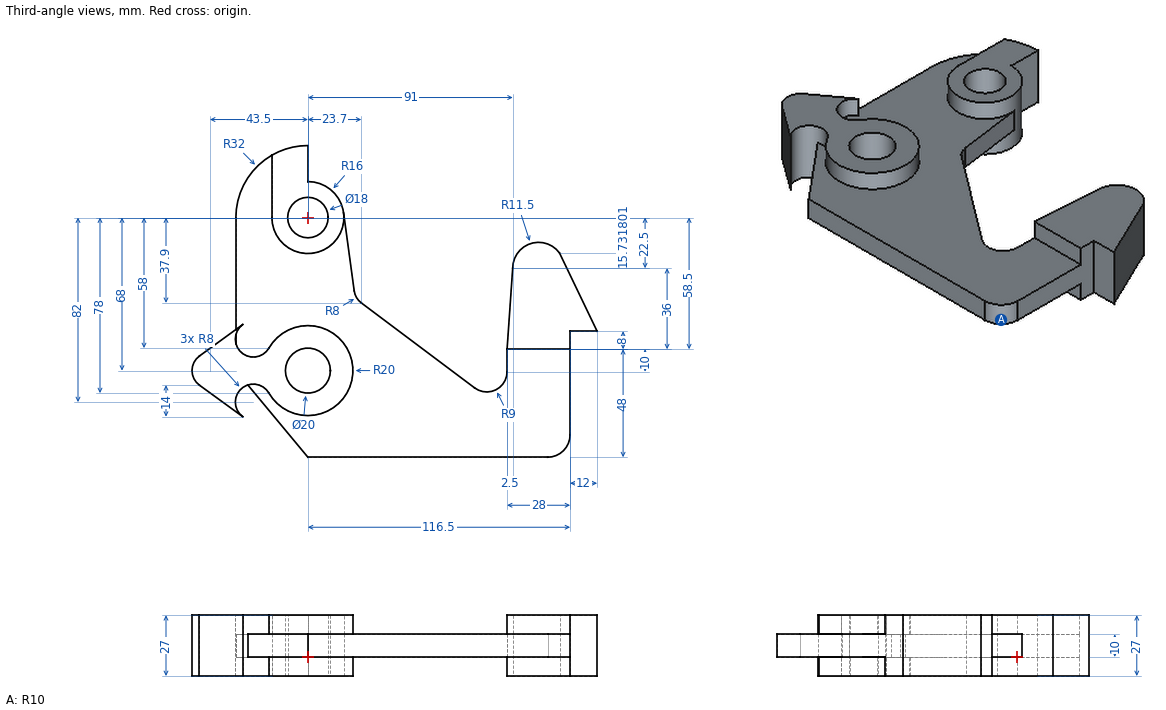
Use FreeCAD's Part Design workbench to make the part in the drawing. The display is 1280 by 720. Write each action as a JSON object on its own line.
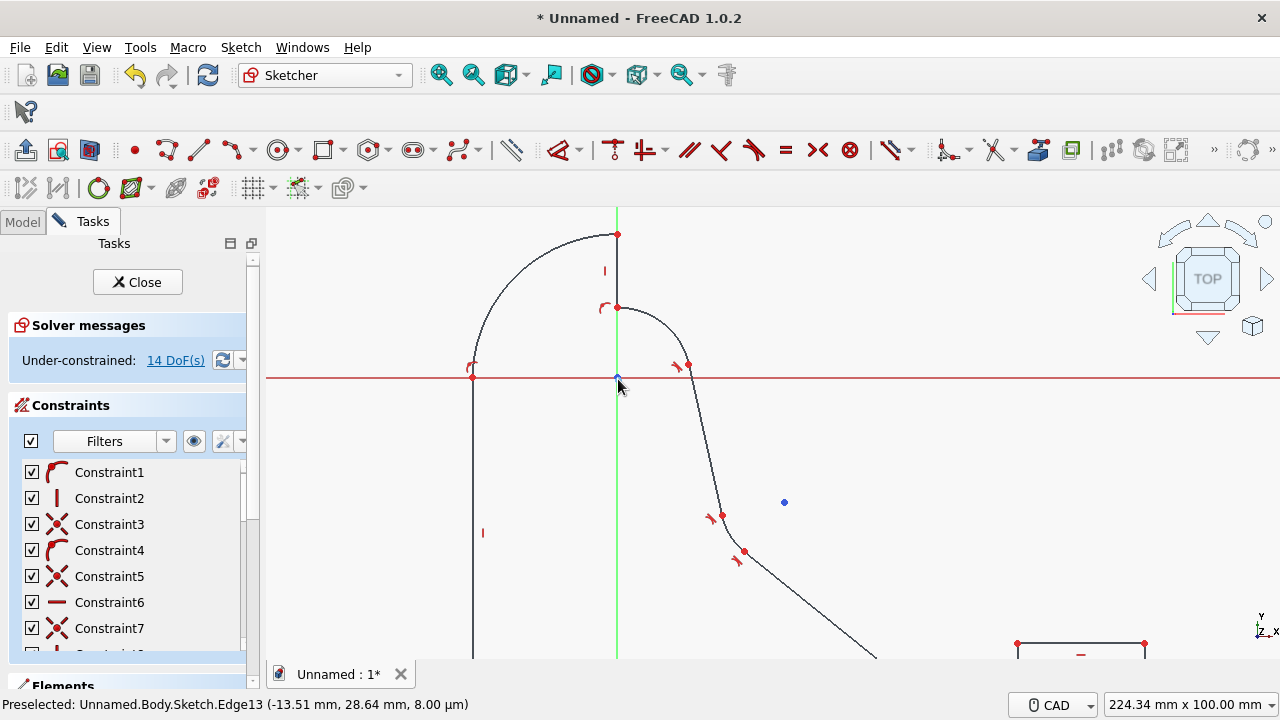
{"action": "left_click_drag", "start_coordinate": [607, 368], "coordinate": [628, 390]}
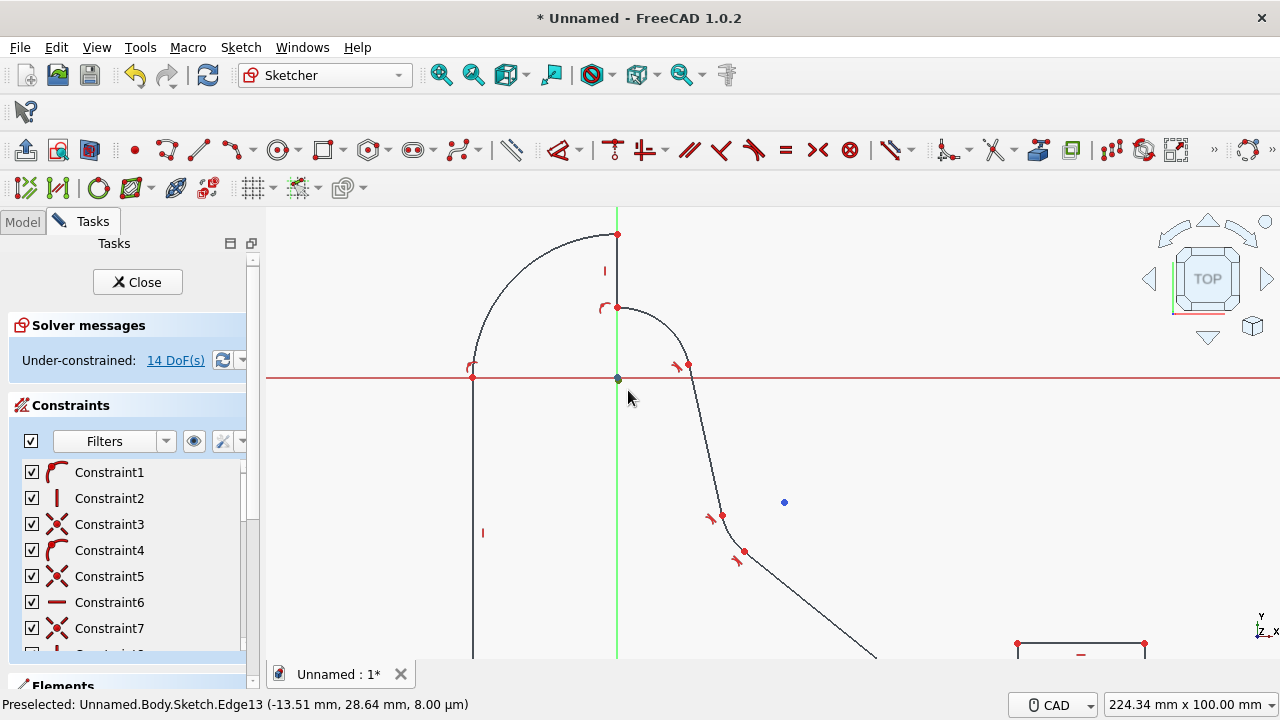
{"action": "left_click", "coordinate": [614, 150]}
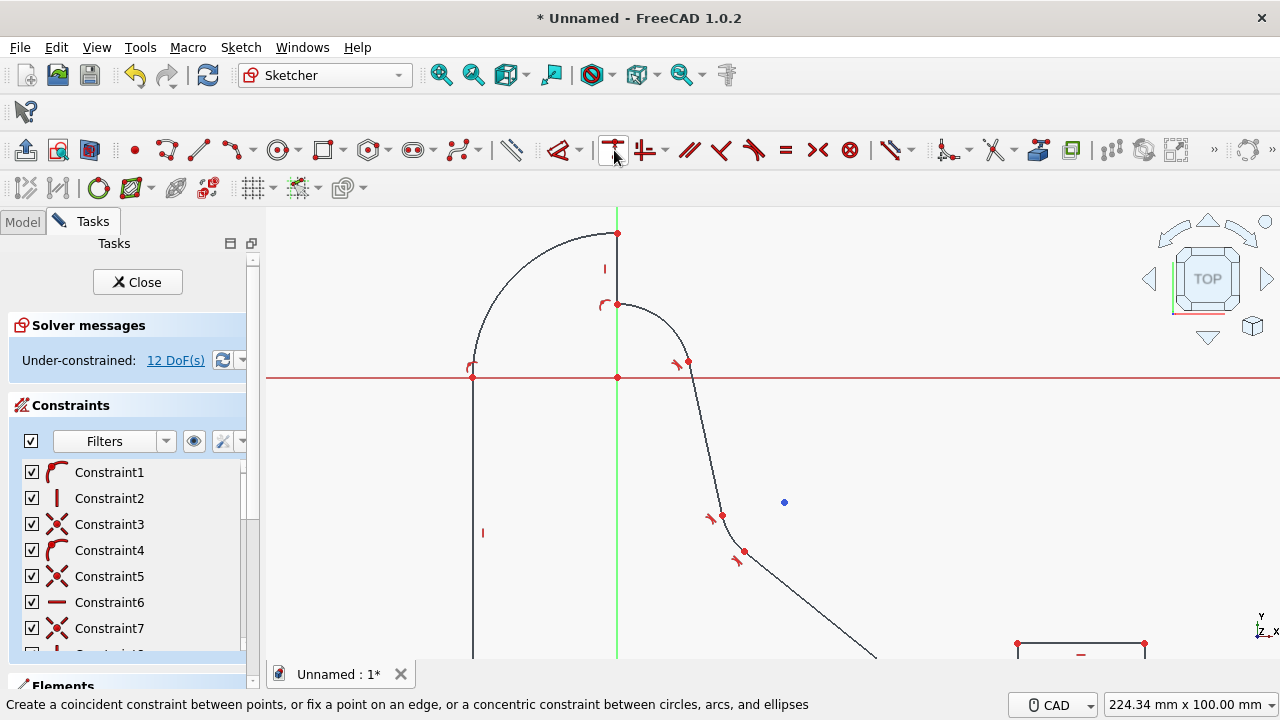
{"action": "scroll", "coordinate": [620, 341], "scroll_direction": "down", "scroll_amount": 4}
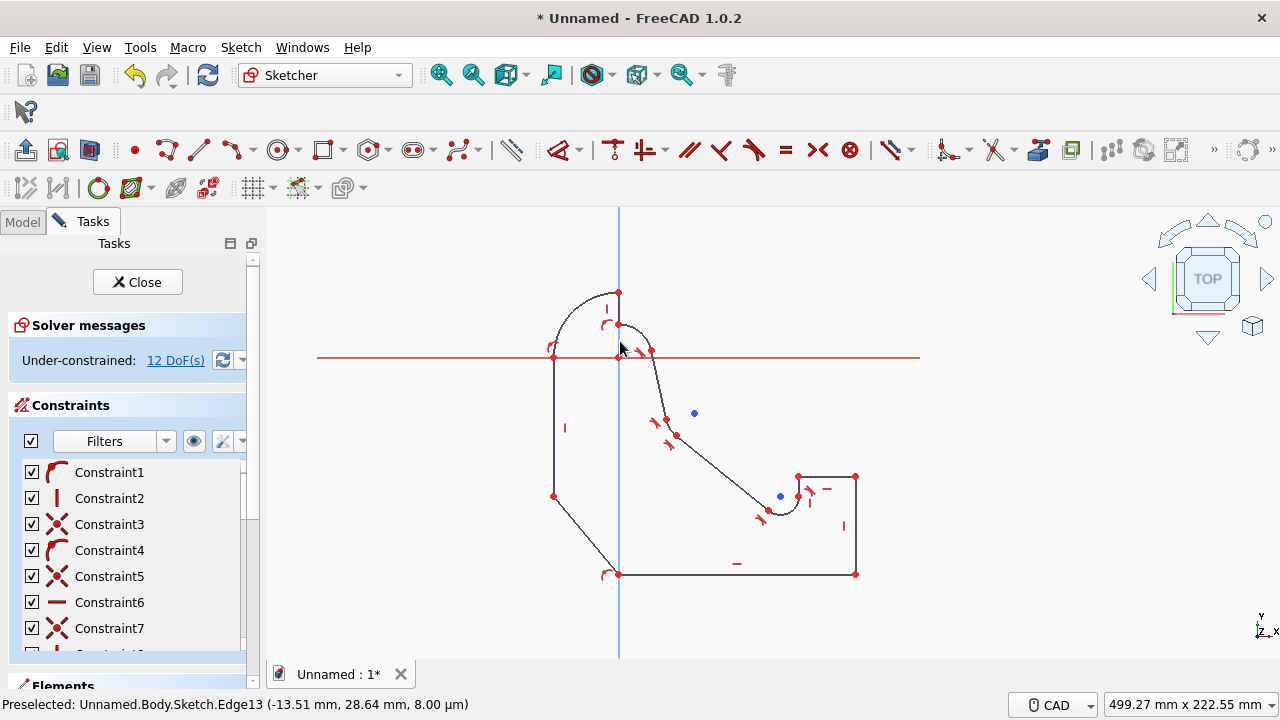
{"action": "scroll", "coordinate": [780, 515], "scroll_direction": "up", "scroll_amount": 4}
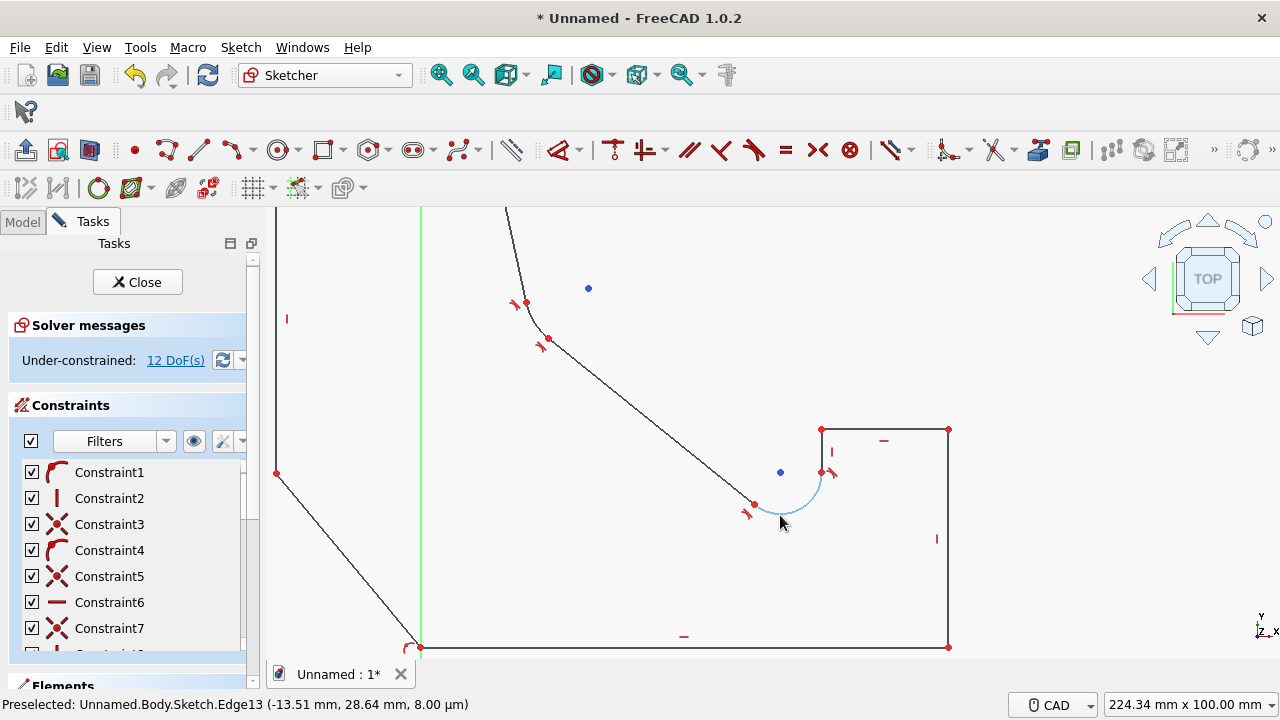
{"action": "left_click", "coordinate": [780, 514]}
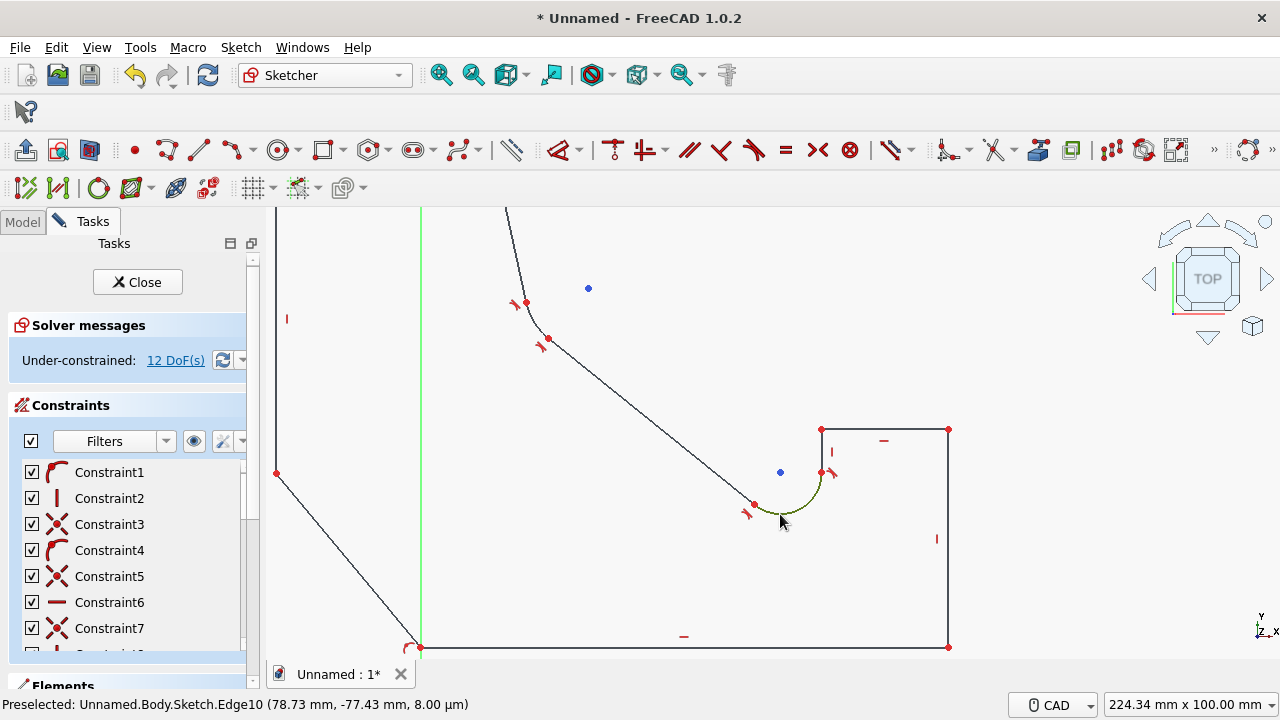
{"action": "left_click", "coordinate": [582, 150]}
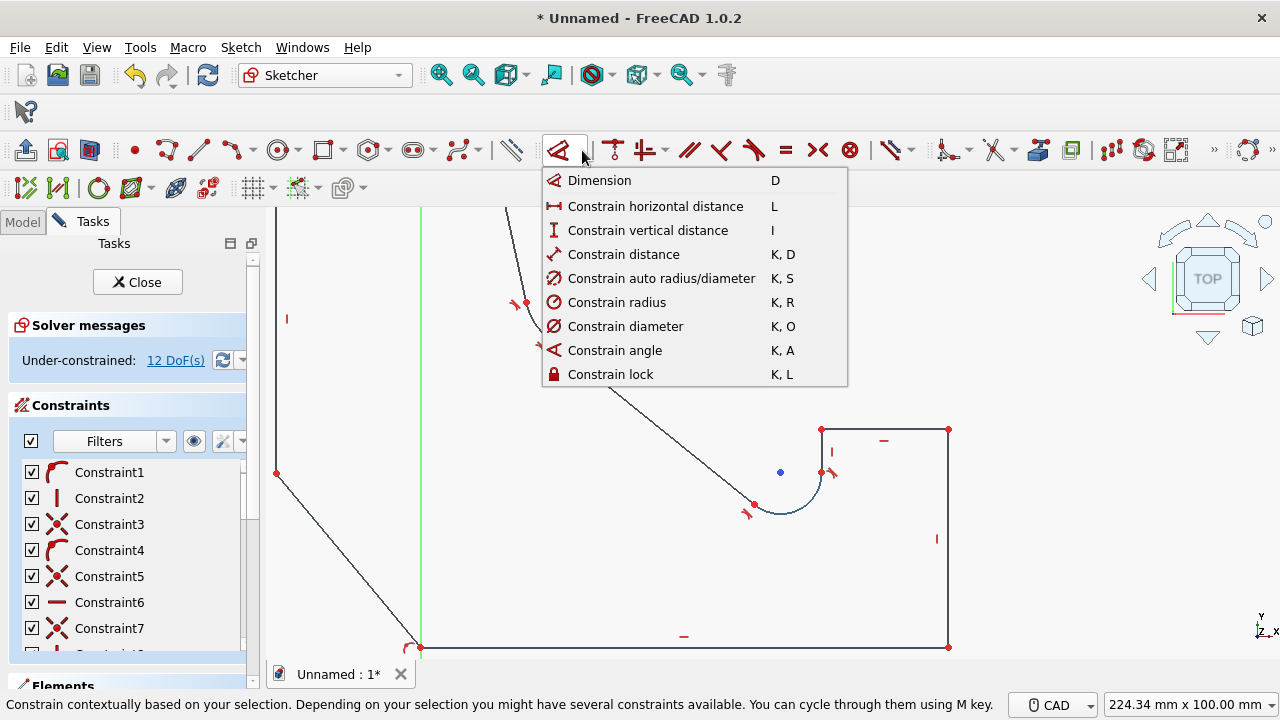
{"action": "left_click", "coordinate": [695, 302]}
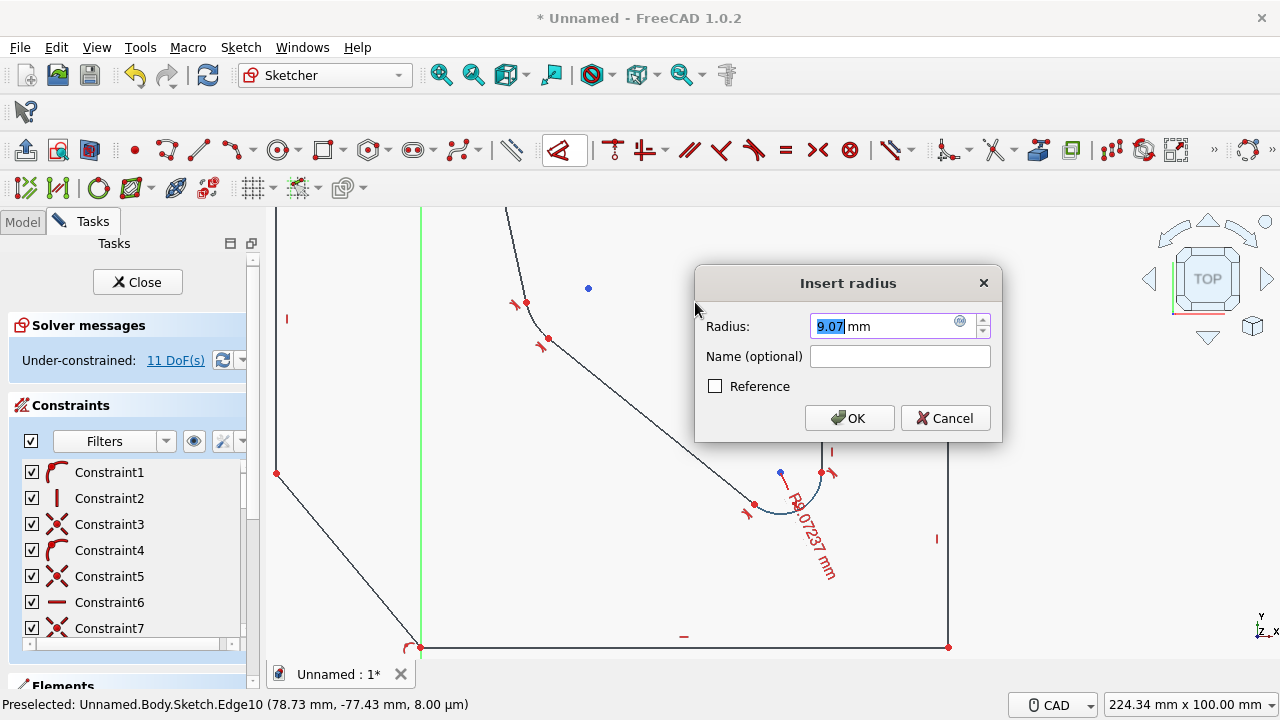
{"action": "type", "text": "9"}
{"action": "key", "text": "Return"}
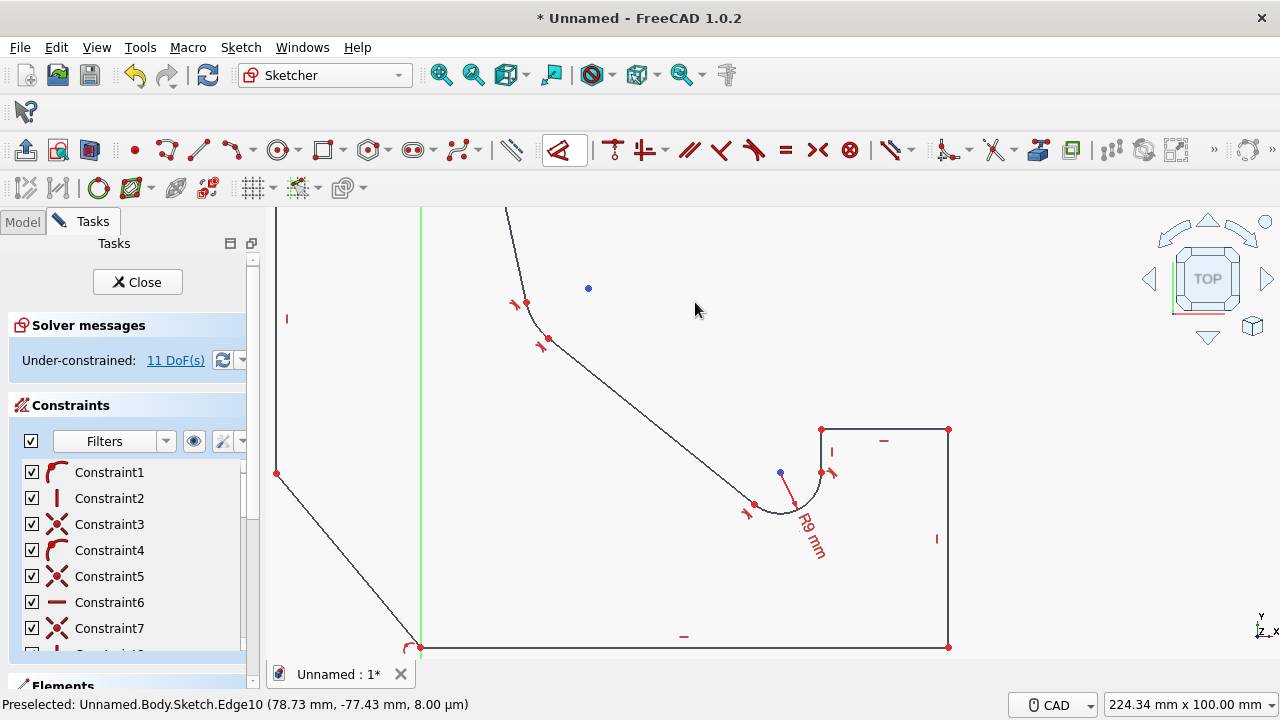
{"action": "left_click", "coordinate": [530, 314]}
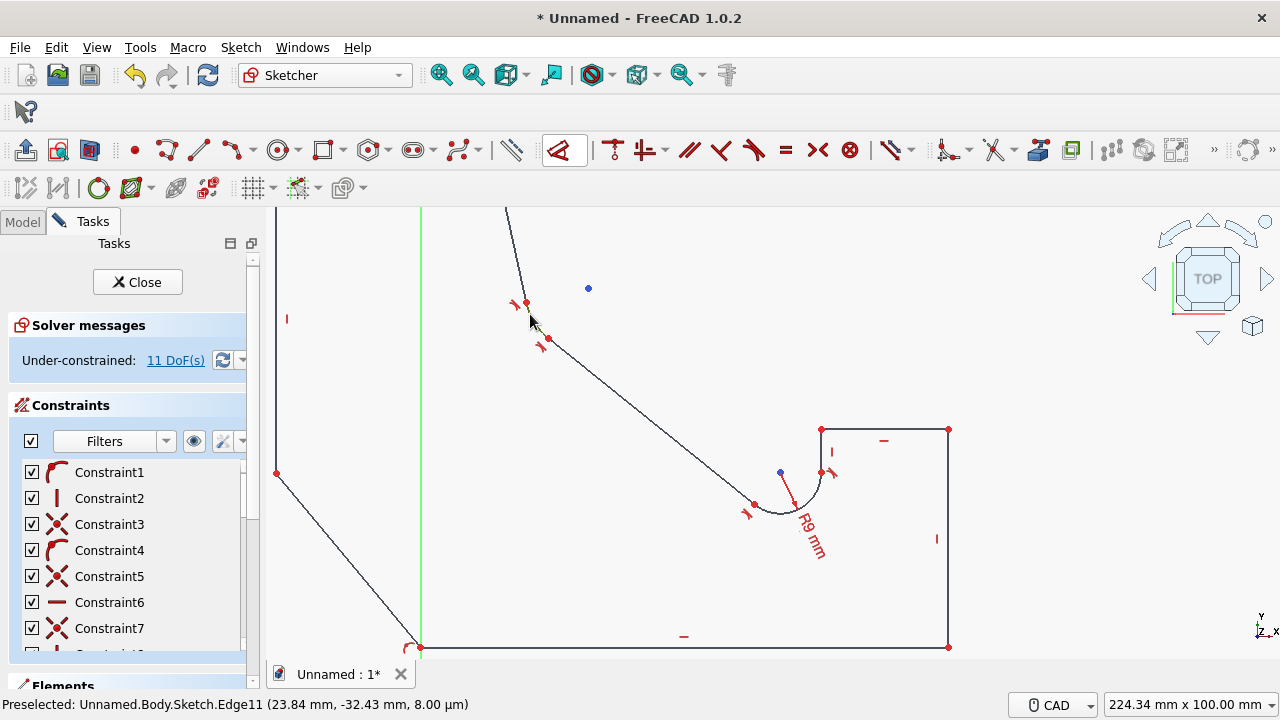
{"action": "key", "text": "k r"}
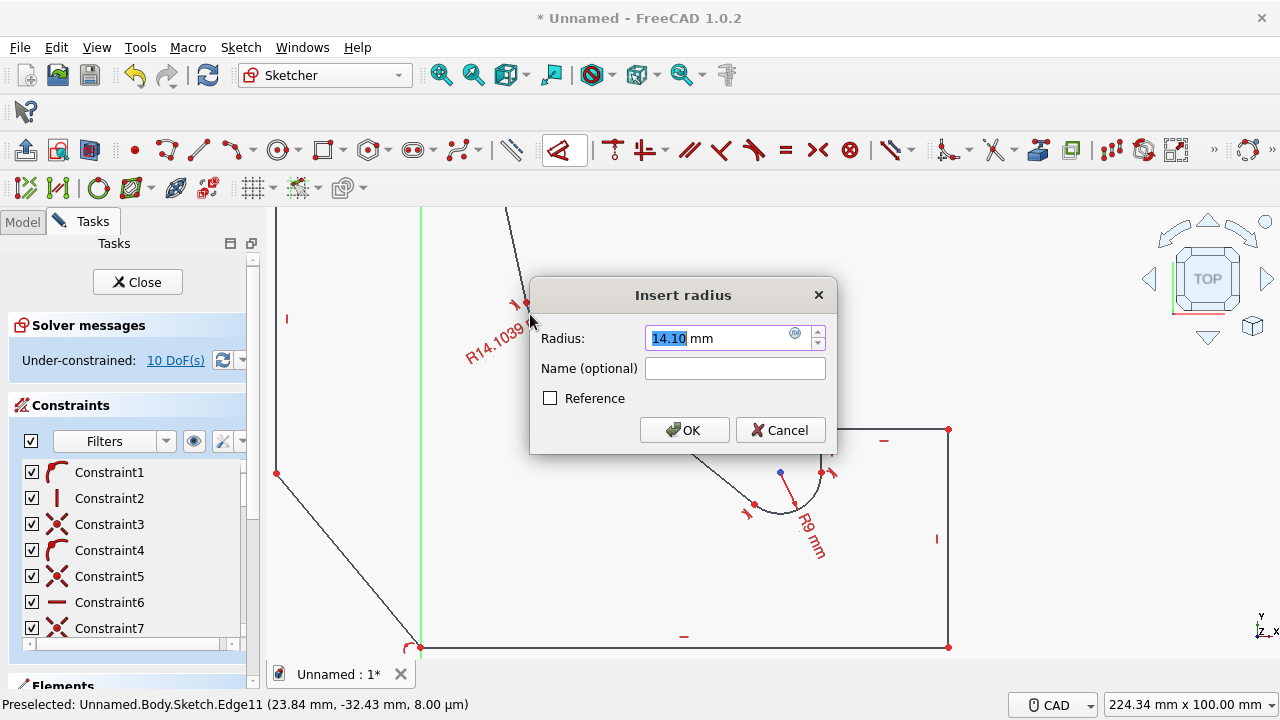
{"action": "type", "text": "8"}
{"action": "key", "text": "Return"}